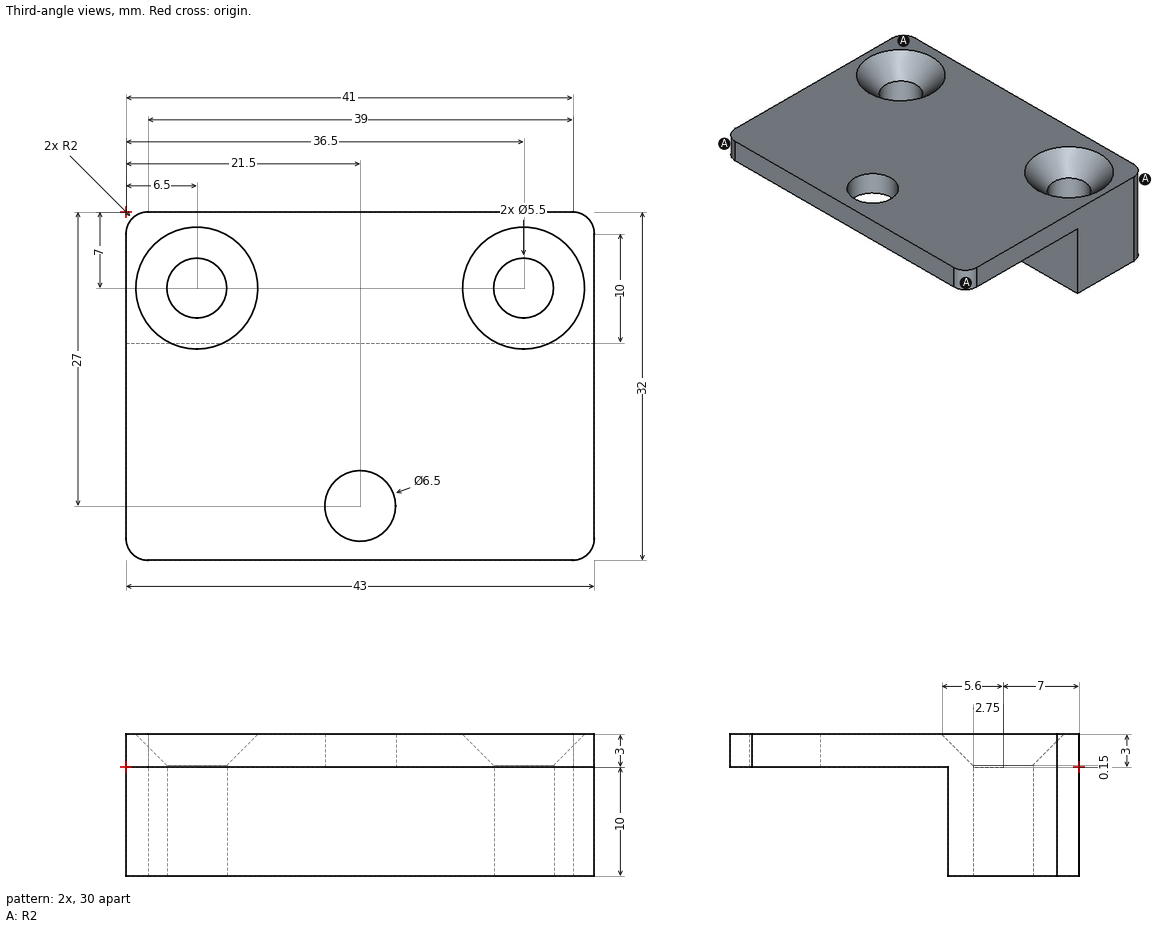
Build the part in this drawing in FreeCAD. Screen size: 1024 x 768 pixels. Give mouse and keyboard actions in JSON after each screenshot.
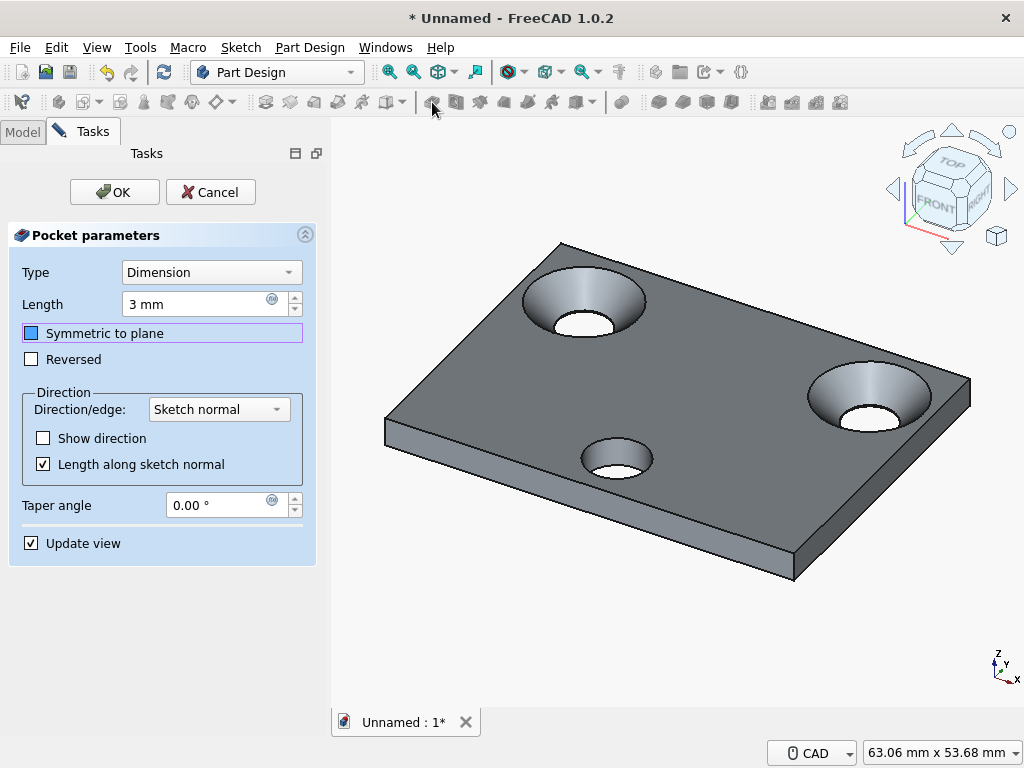
{"action": "left_click", "coordinate": [115, 192]}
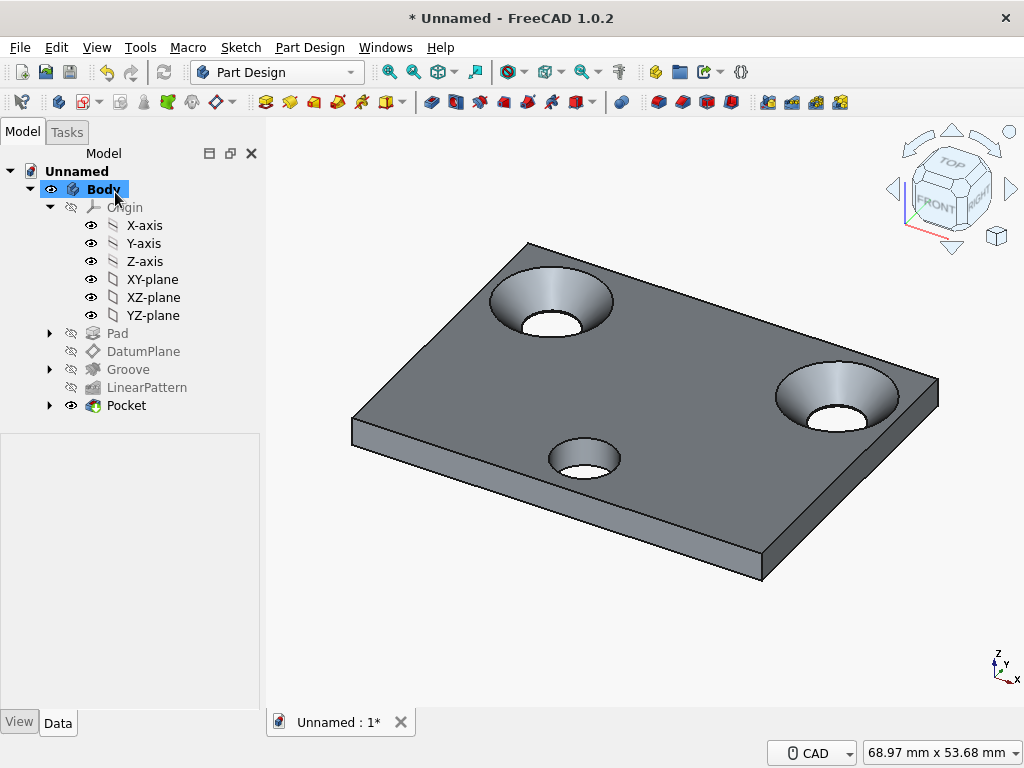
{"action": "left_click", "coordinate": [762, 566]}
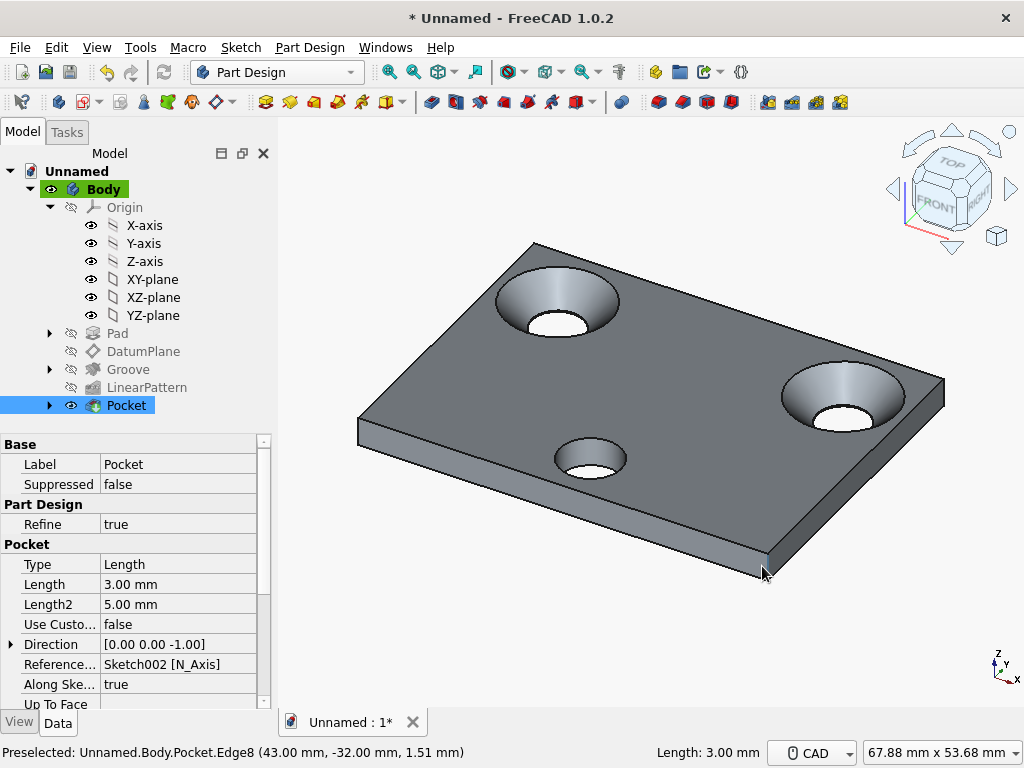
{"action": "key", "text": "0"}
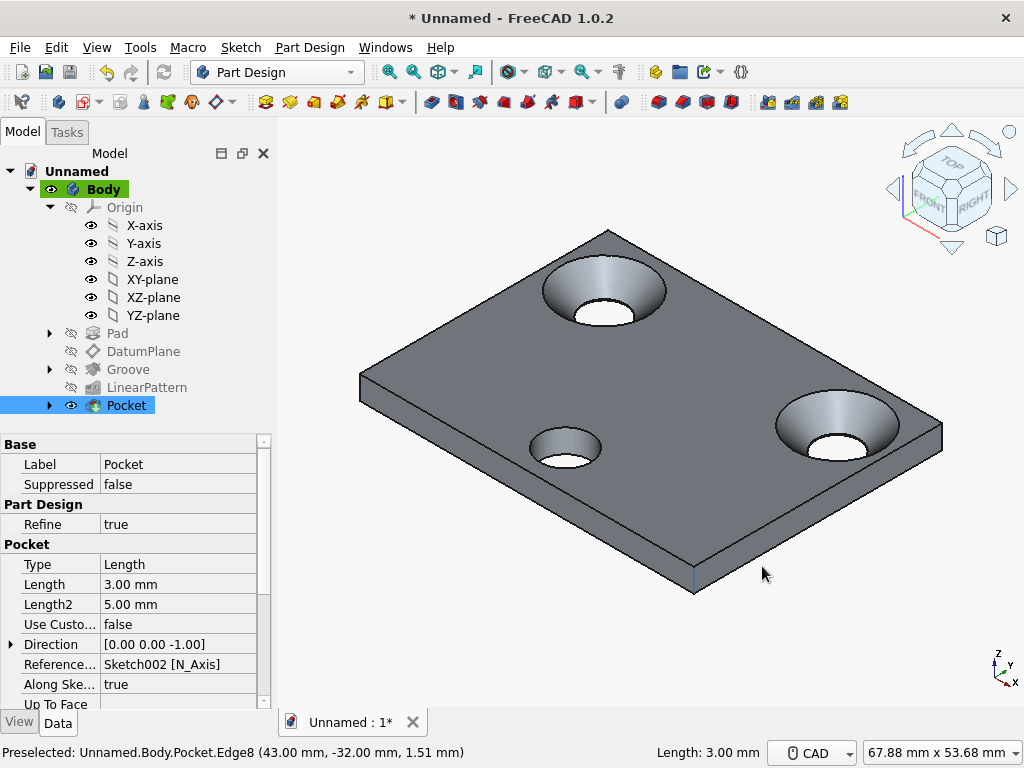
{"action": "key", "text": "2"}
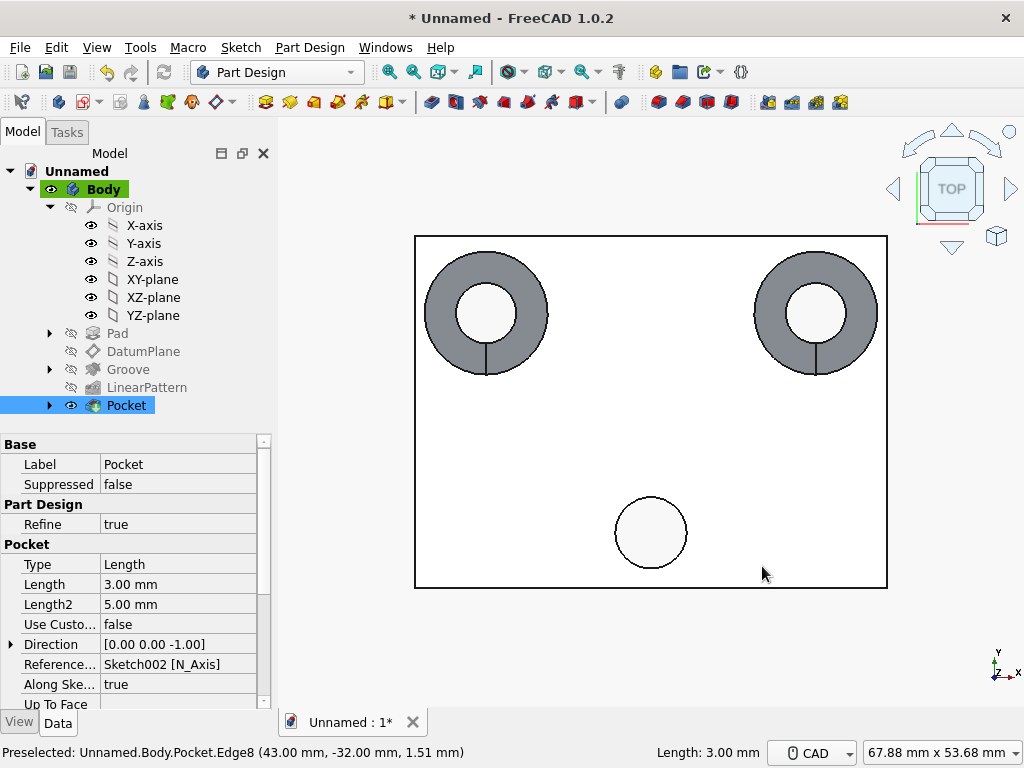
{"action": "key", "text": "1"}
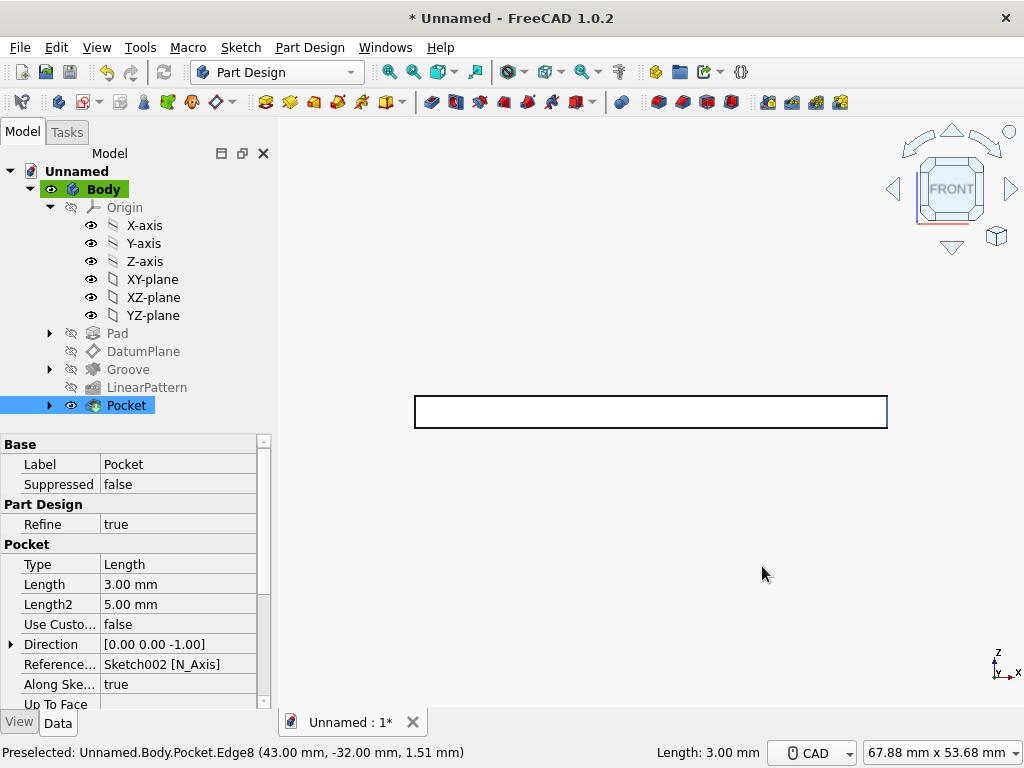
{"action": "left_click", "coordinate": [415, 411], "text": "ctrl"}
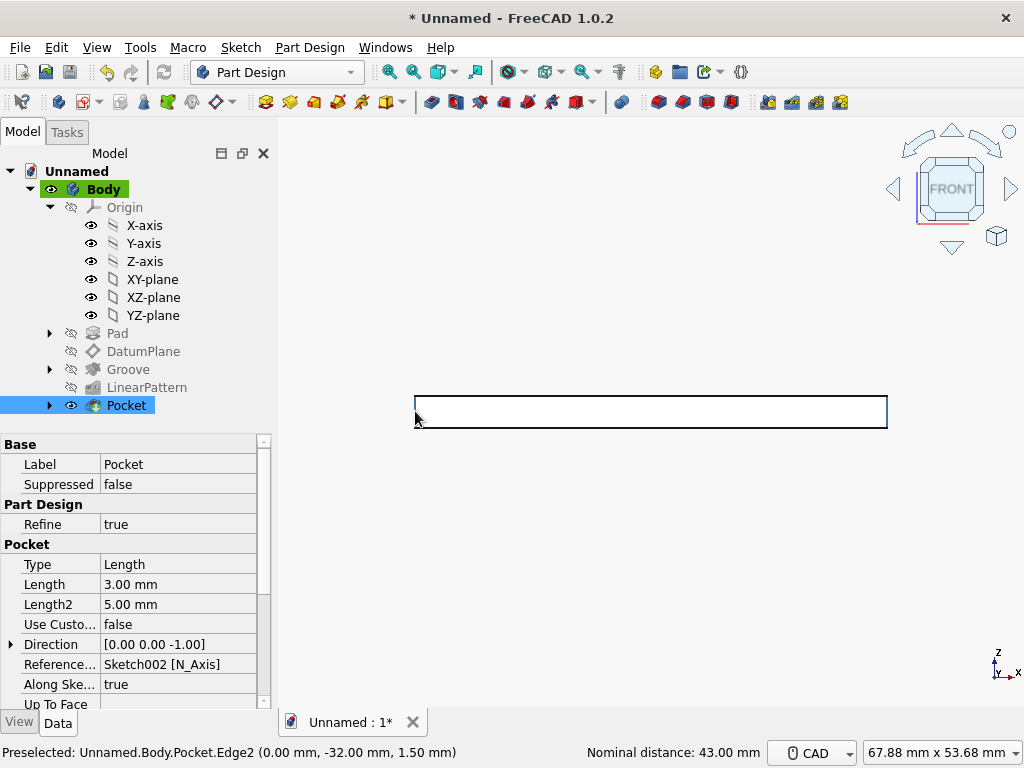
{"action": "key", "text": "3"}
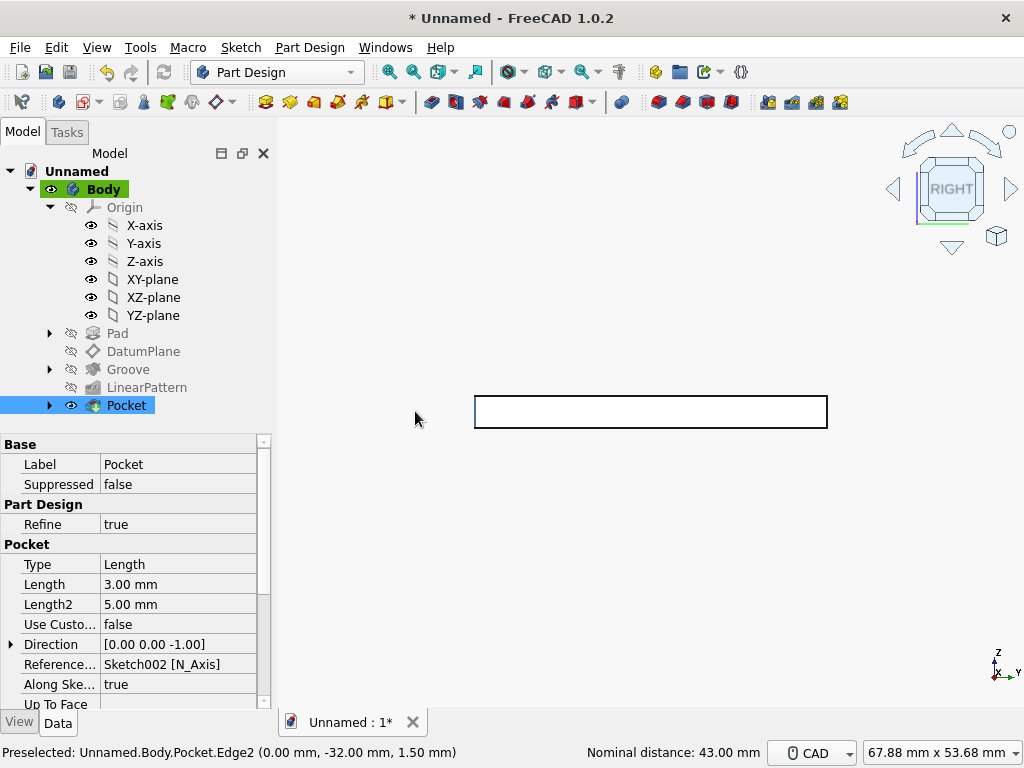
{"action": "left_click", "coordinate": [827, 411], "text": "ctrl"}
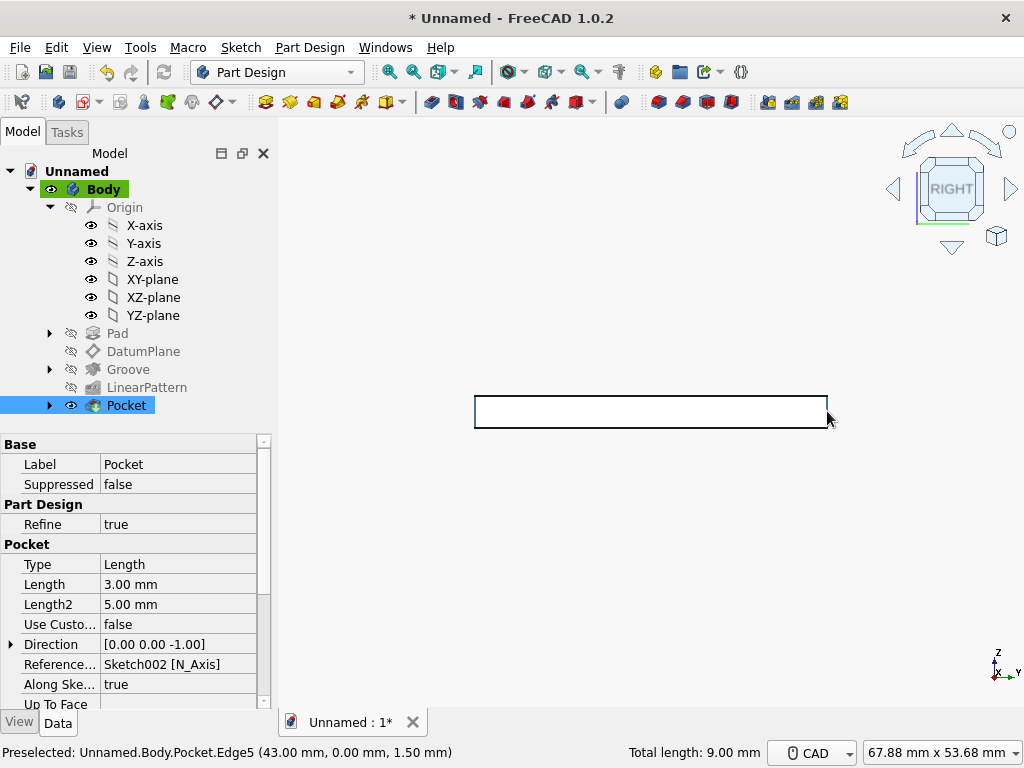
{"action": "key", "text": "5"}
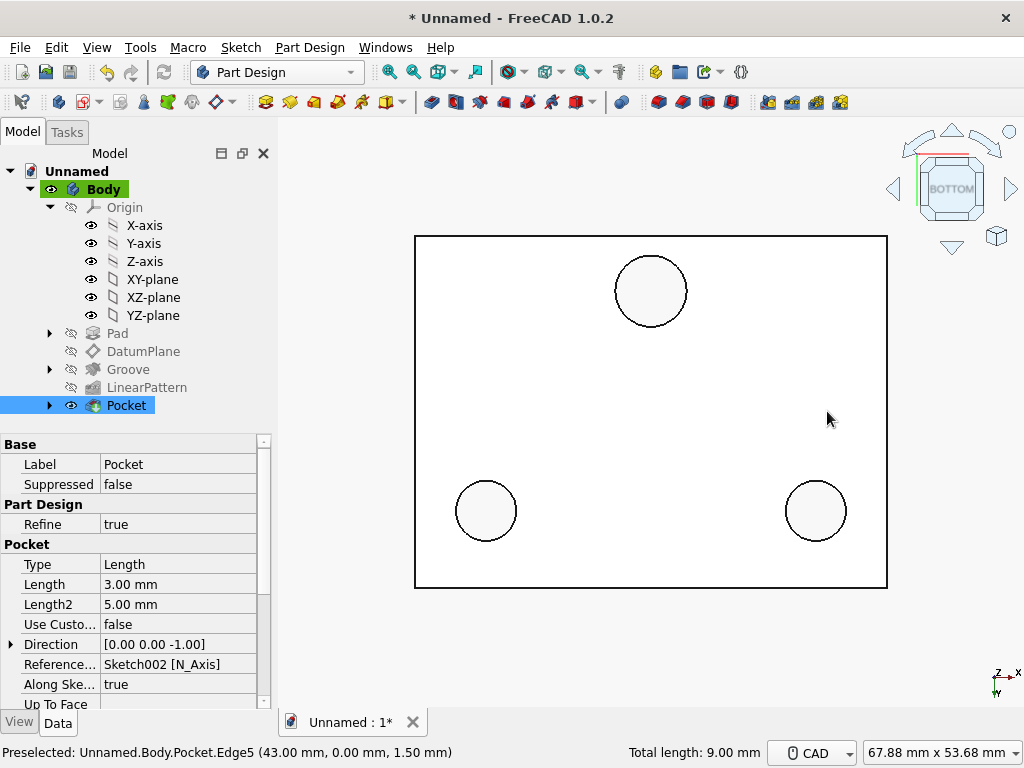
{"action": "key", "text": "4"}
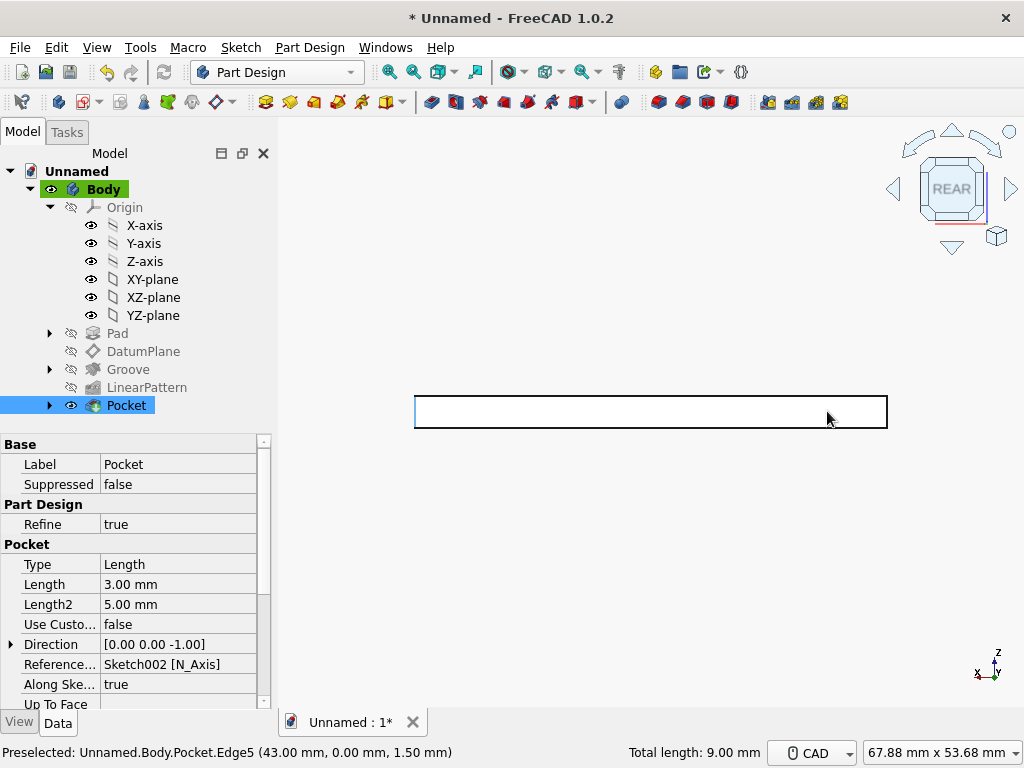
{"action": "left_click", "coordinate": [887, 411], "text": "ctrl"}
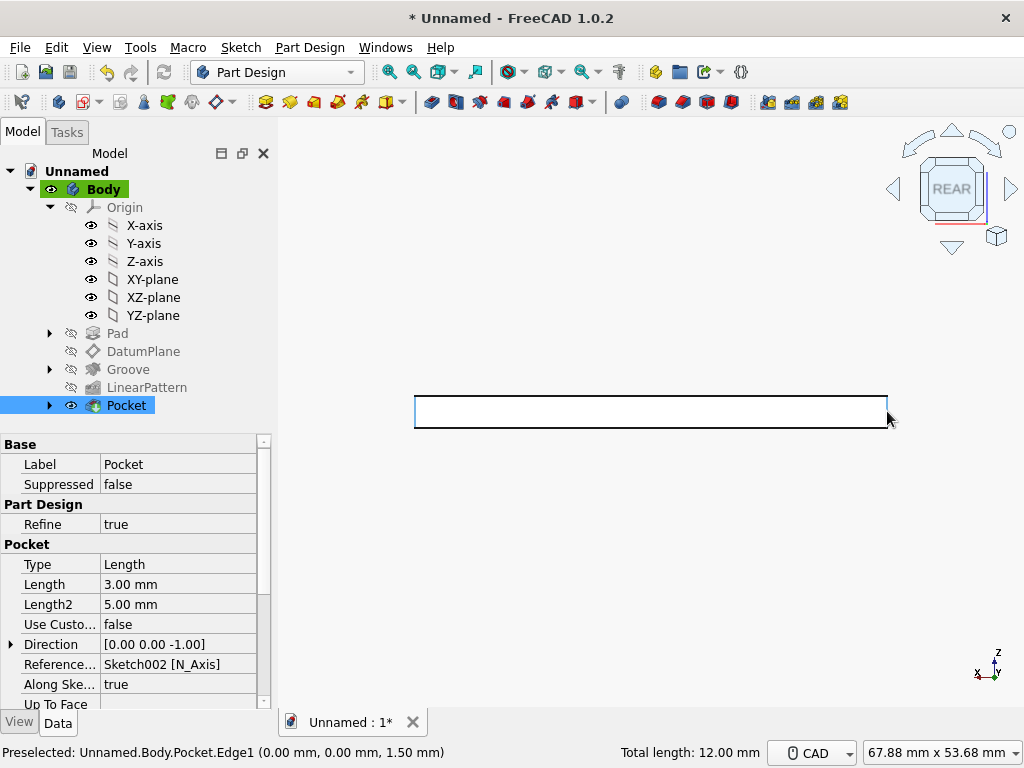
{"action": "left_click", "coordinate": [660, 102]}